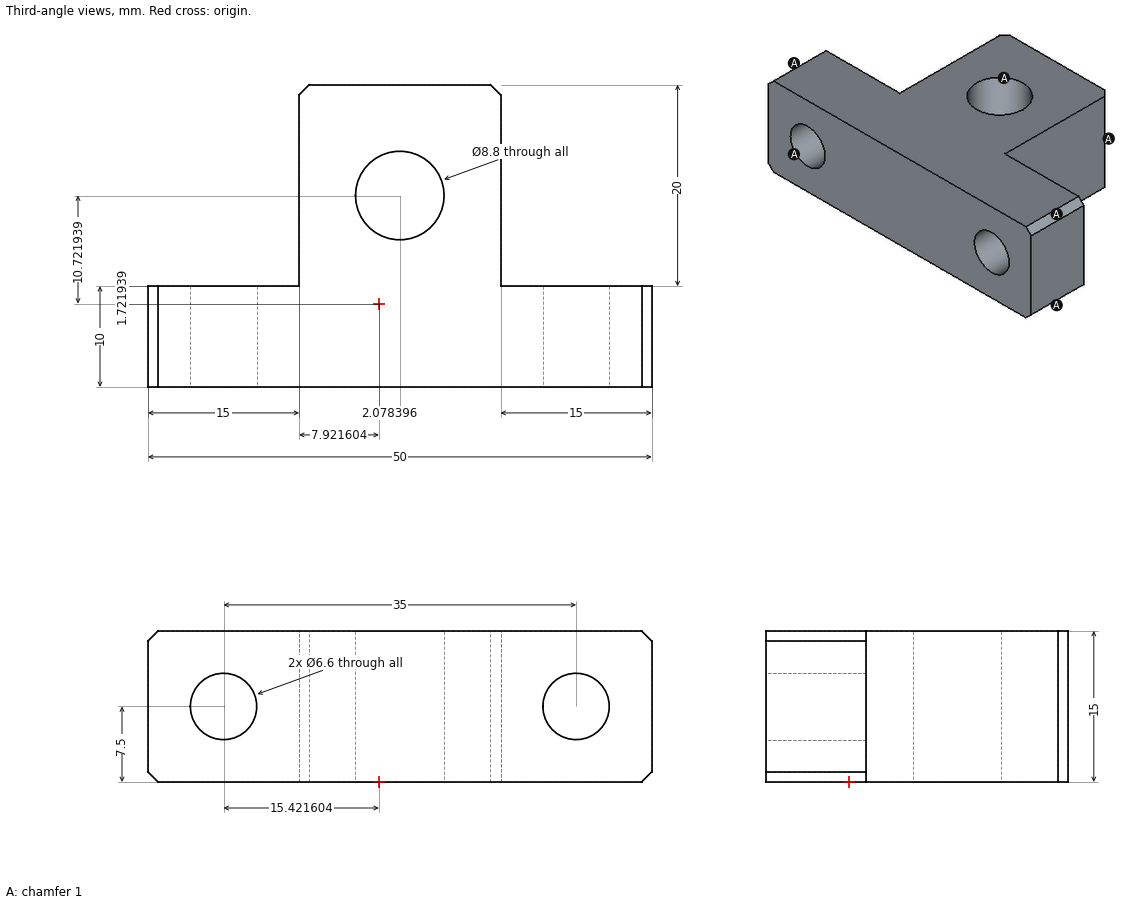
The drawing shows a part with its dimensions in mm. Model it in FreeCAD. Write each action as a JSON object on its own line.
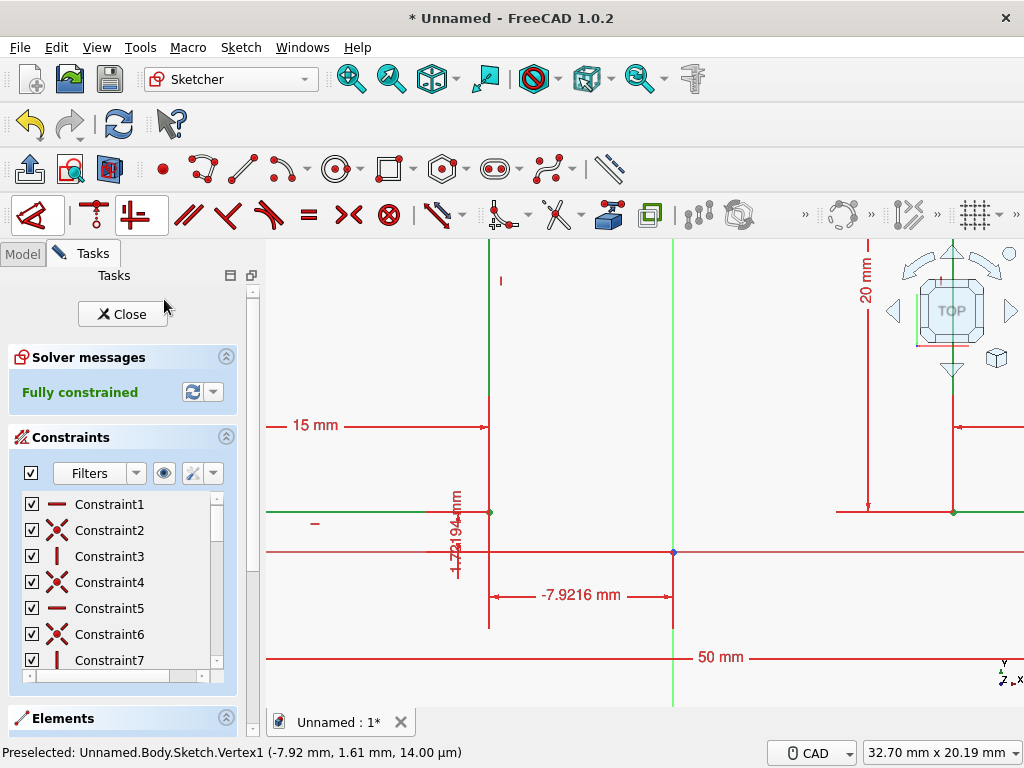
{"action": "left_click", "coordinate": [123, 314]}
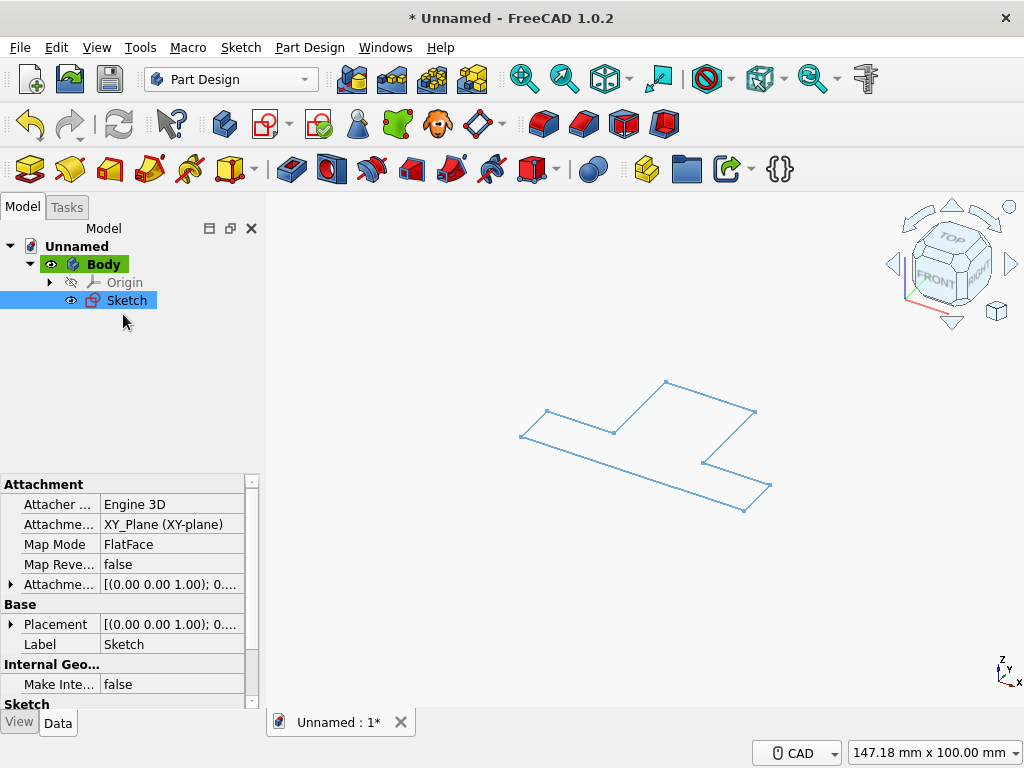
{"action": "left_click", "coordinate": [30, 170]}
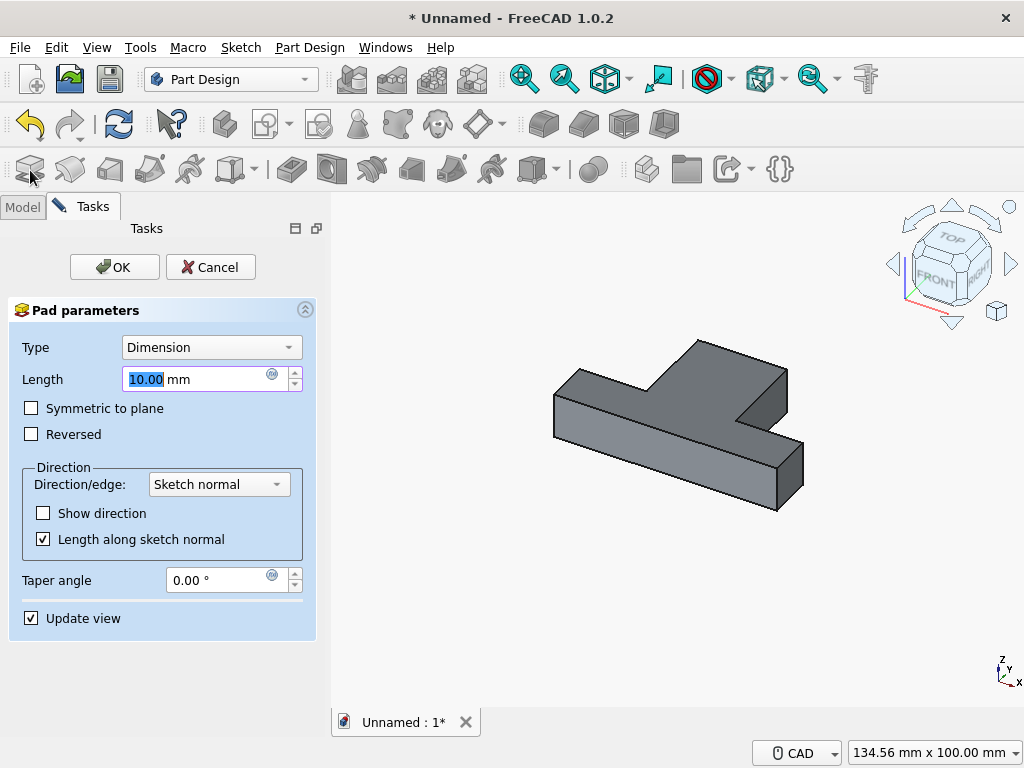
{"action": "type", "text": "15"}
{"action": "key", "text": "Tab"}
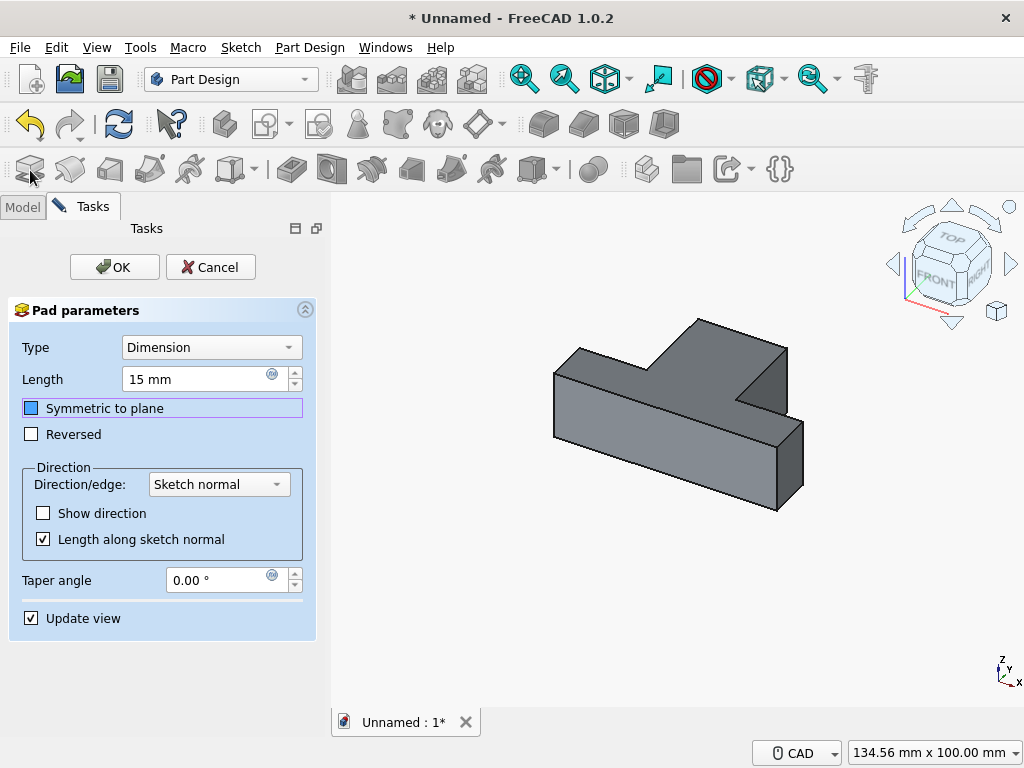
{"action": "left_click", "coordinate": [115, 267]}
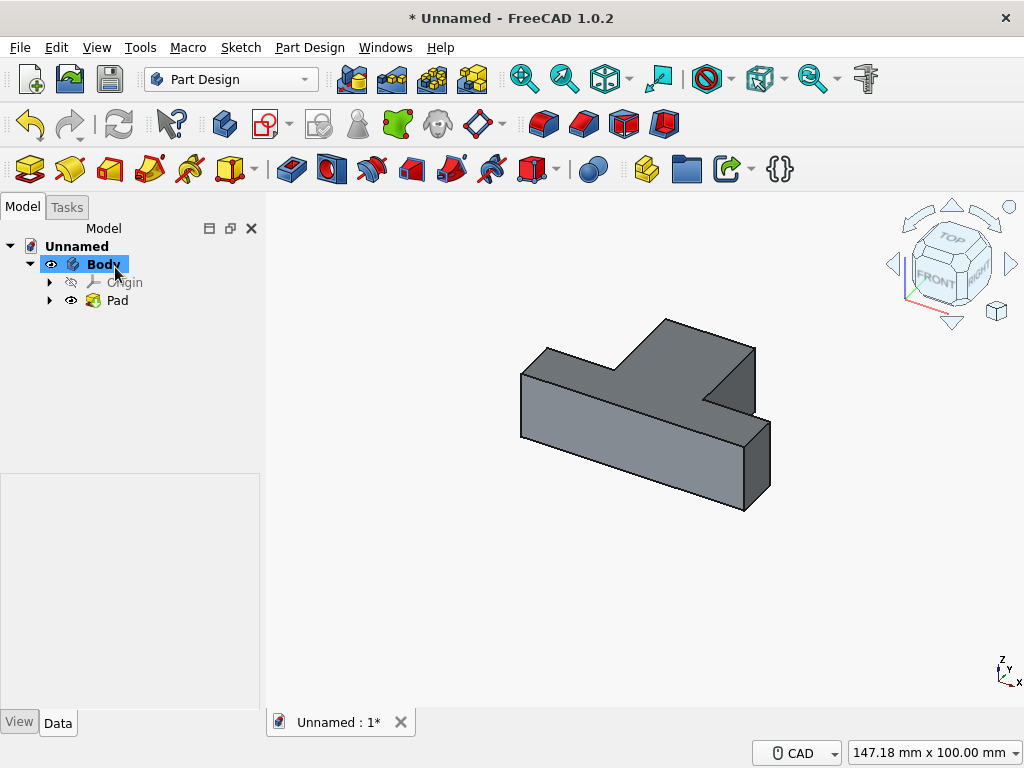
{"action": "key", "text": "v f"}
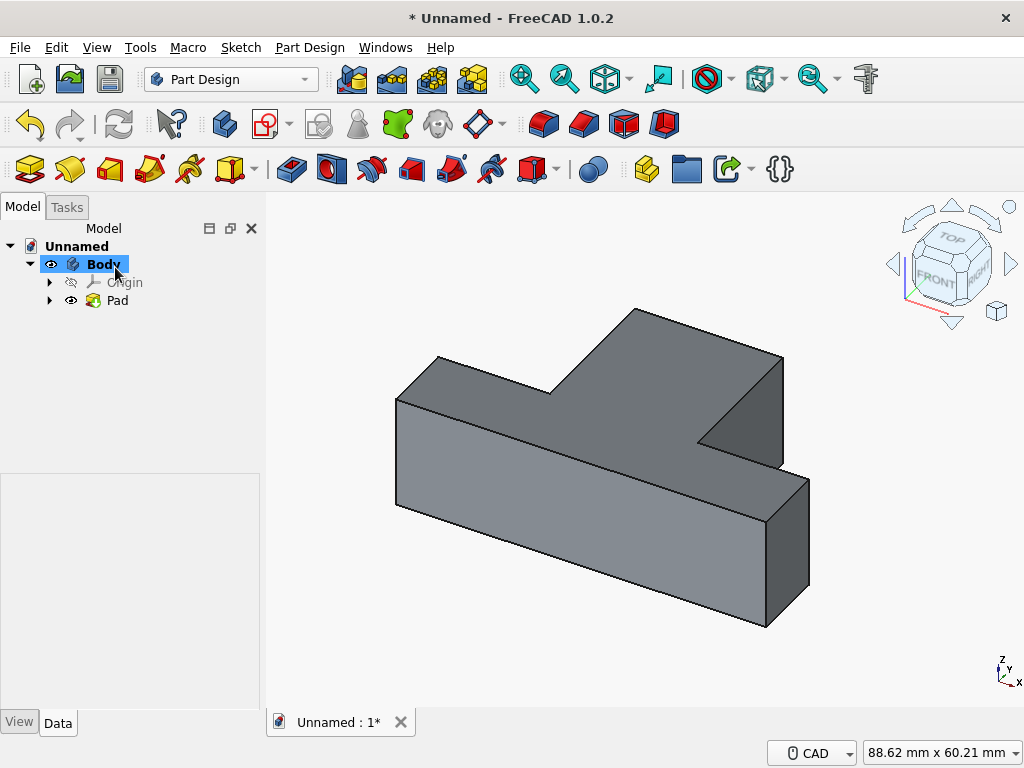
{"action": "left_click", "coordinate": [787, 500]}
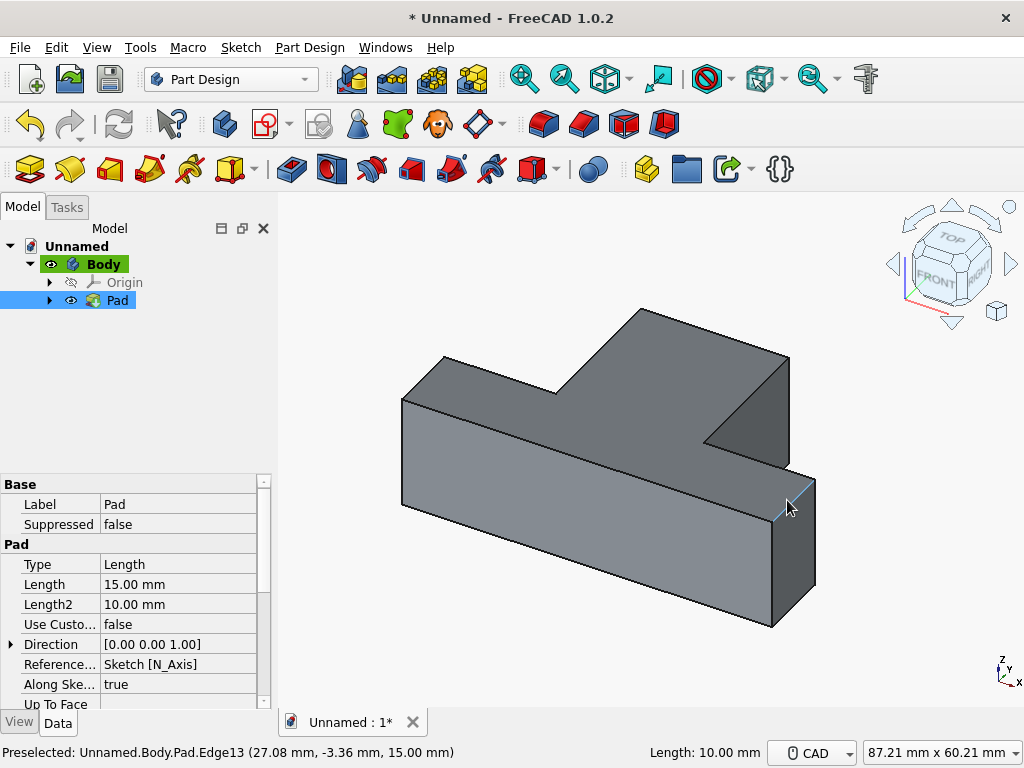
{"action": "key", "text": "0"}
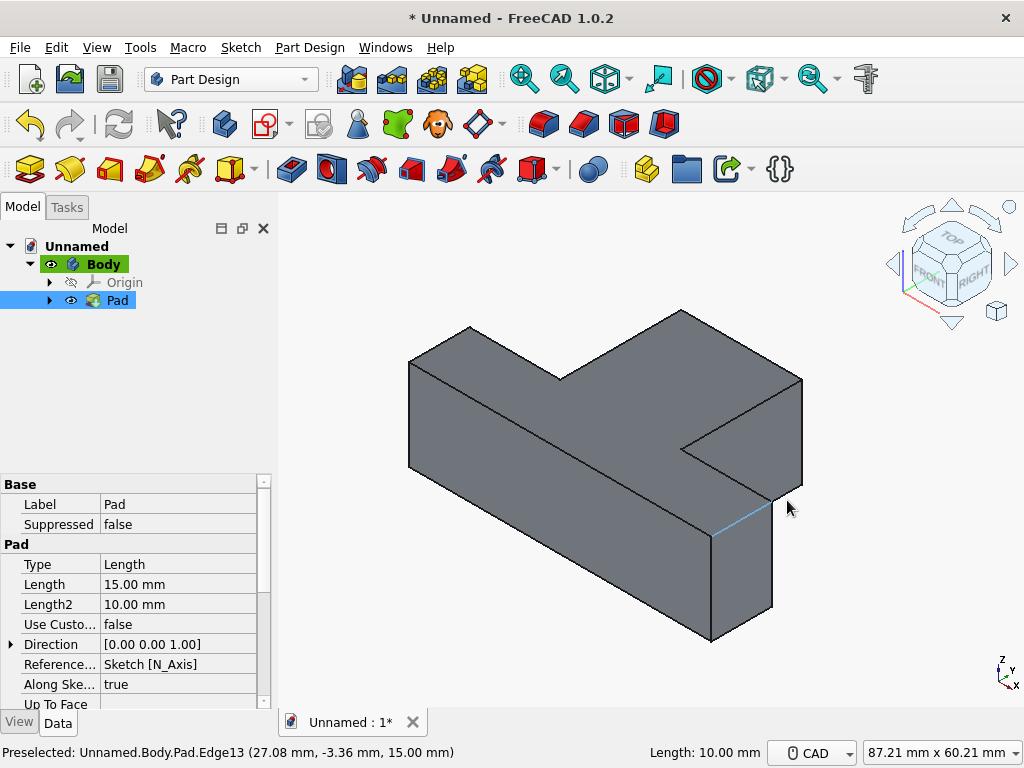
{"action": "key", "text": "2"}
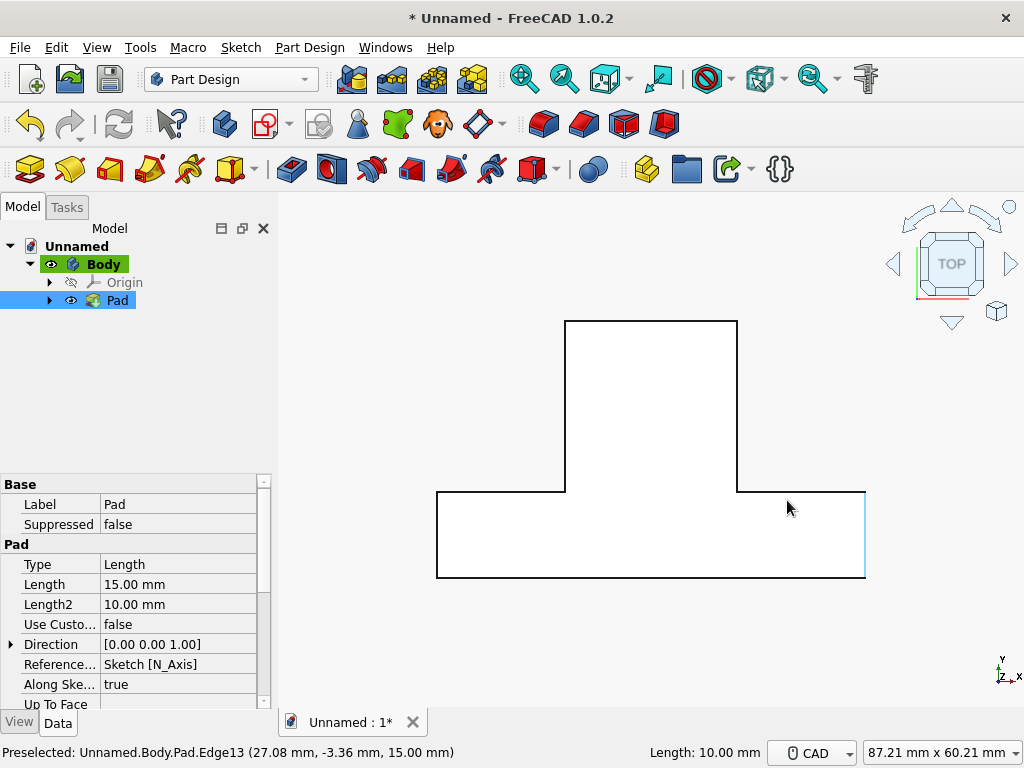
{"action": "left_click", "coordinate": [437, 534], "text": "ctrl"}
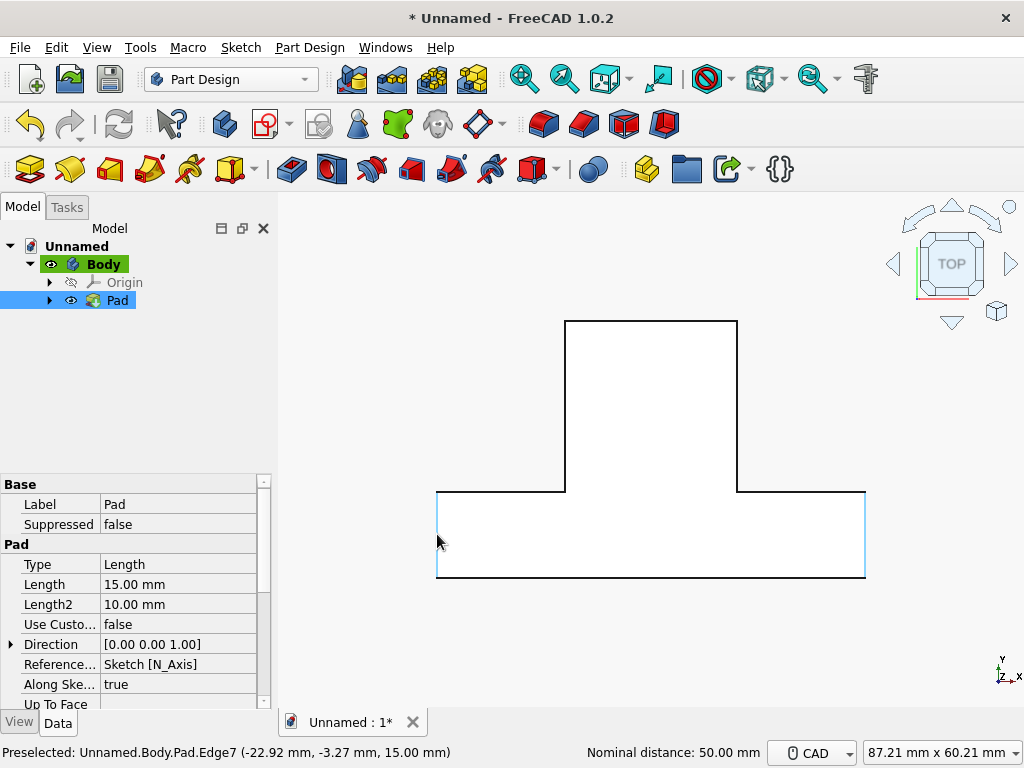
{"action": "key", "text": "1"}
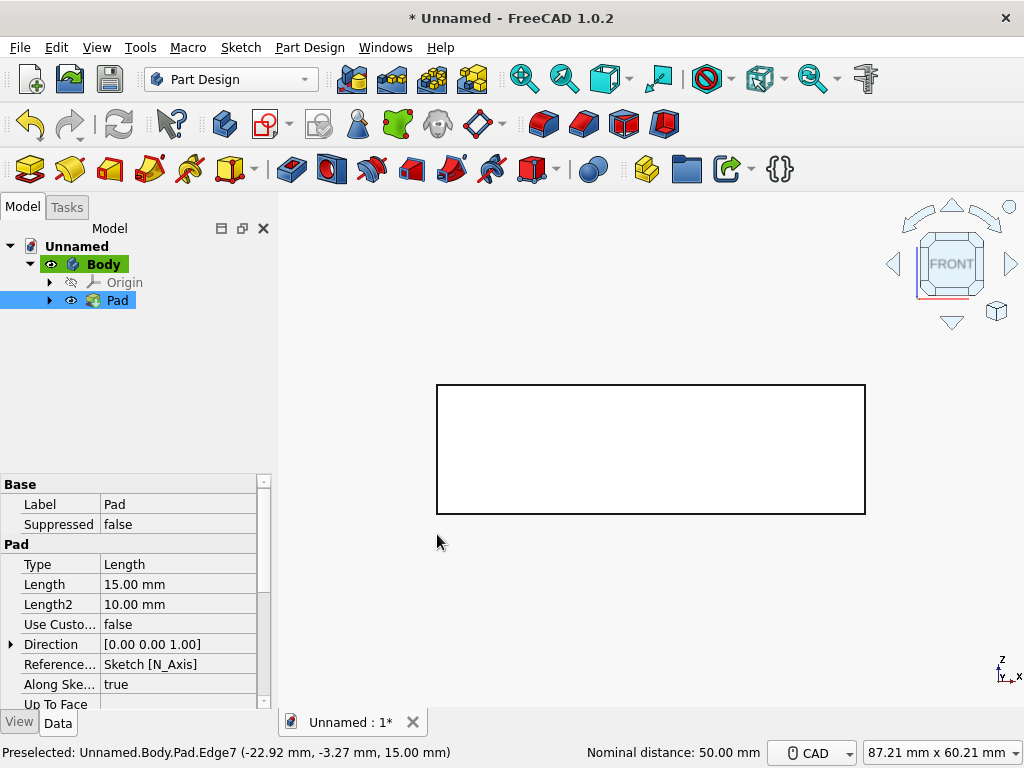
{"action": "key", "text": "3"}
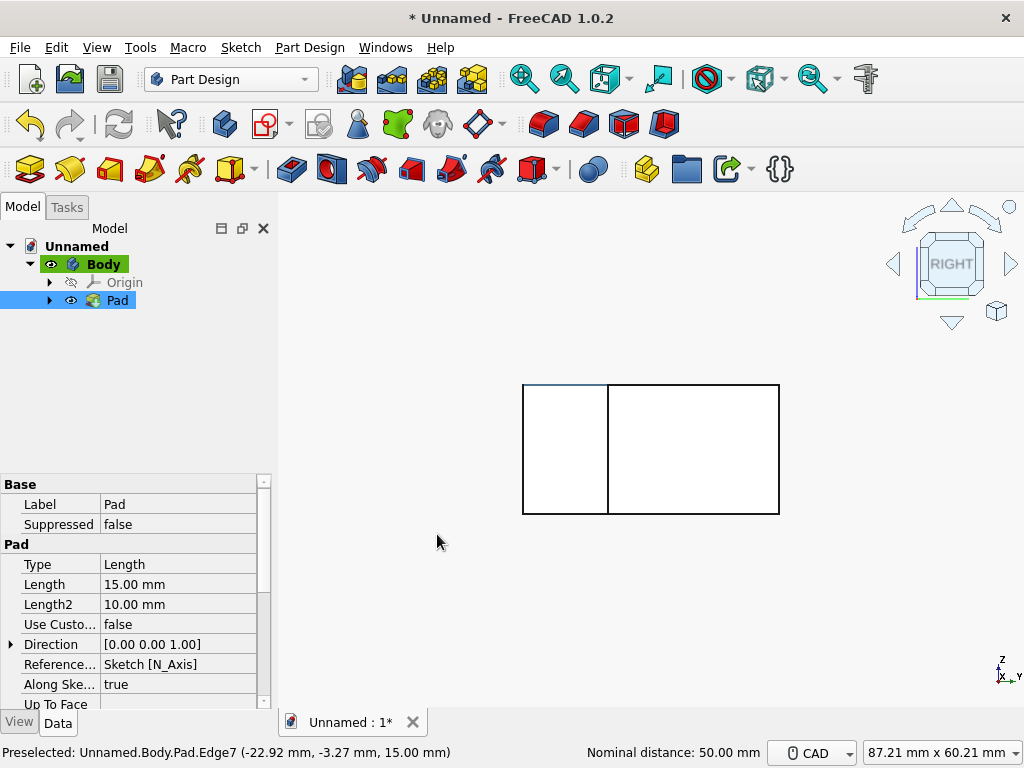
{"action": "left_click", "coordinate": [526, 80]}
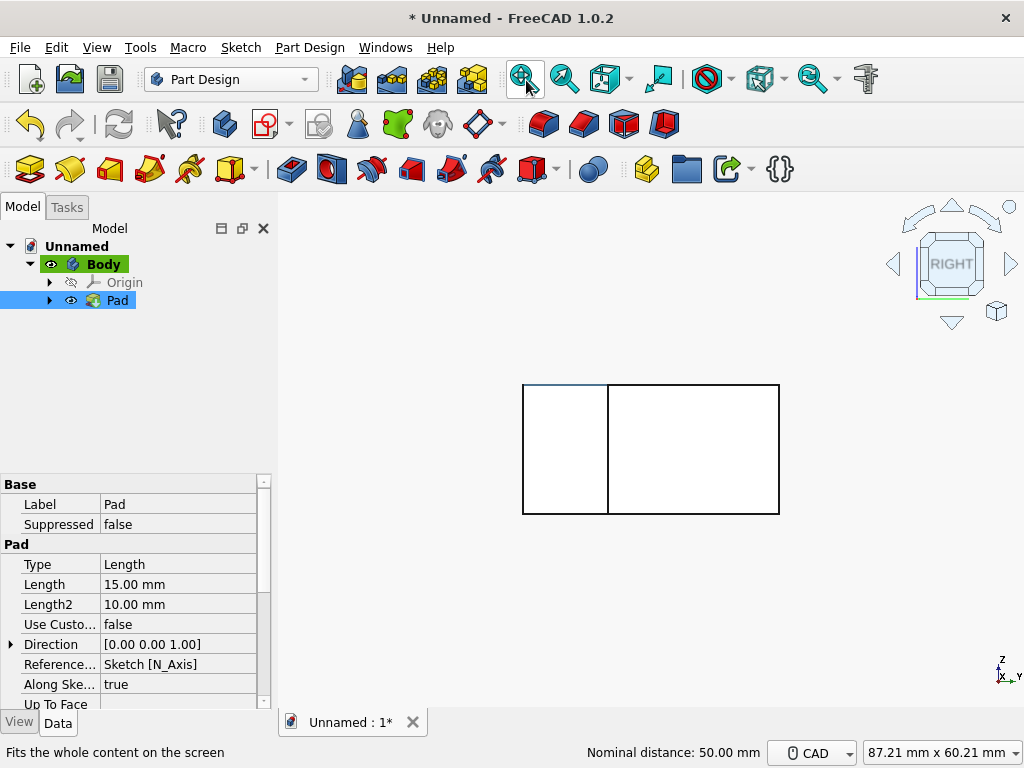
{"action": "left_click", "coordinate": [779, 448], "text": "ctrl"}